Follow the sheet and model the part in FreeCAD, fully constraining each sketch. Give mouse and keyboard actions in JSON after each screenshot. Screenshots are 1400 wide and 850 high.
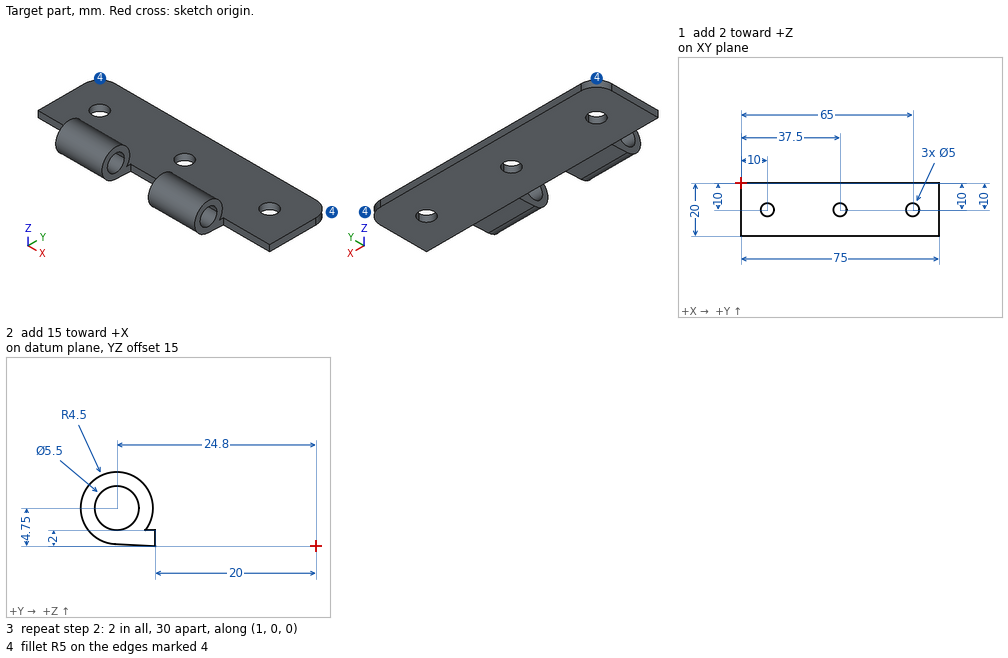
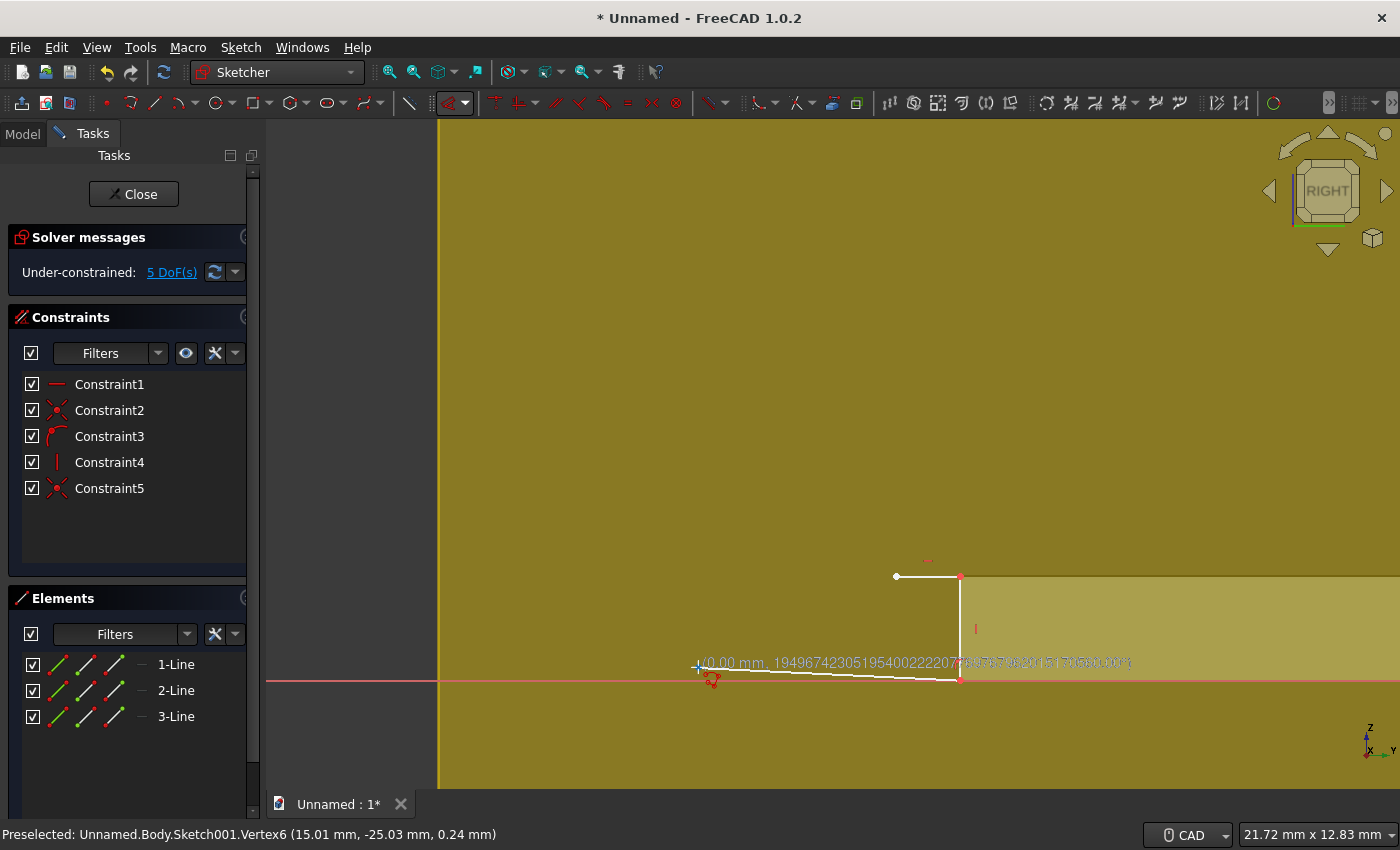
{"action": "key", "text": "g 3 a"}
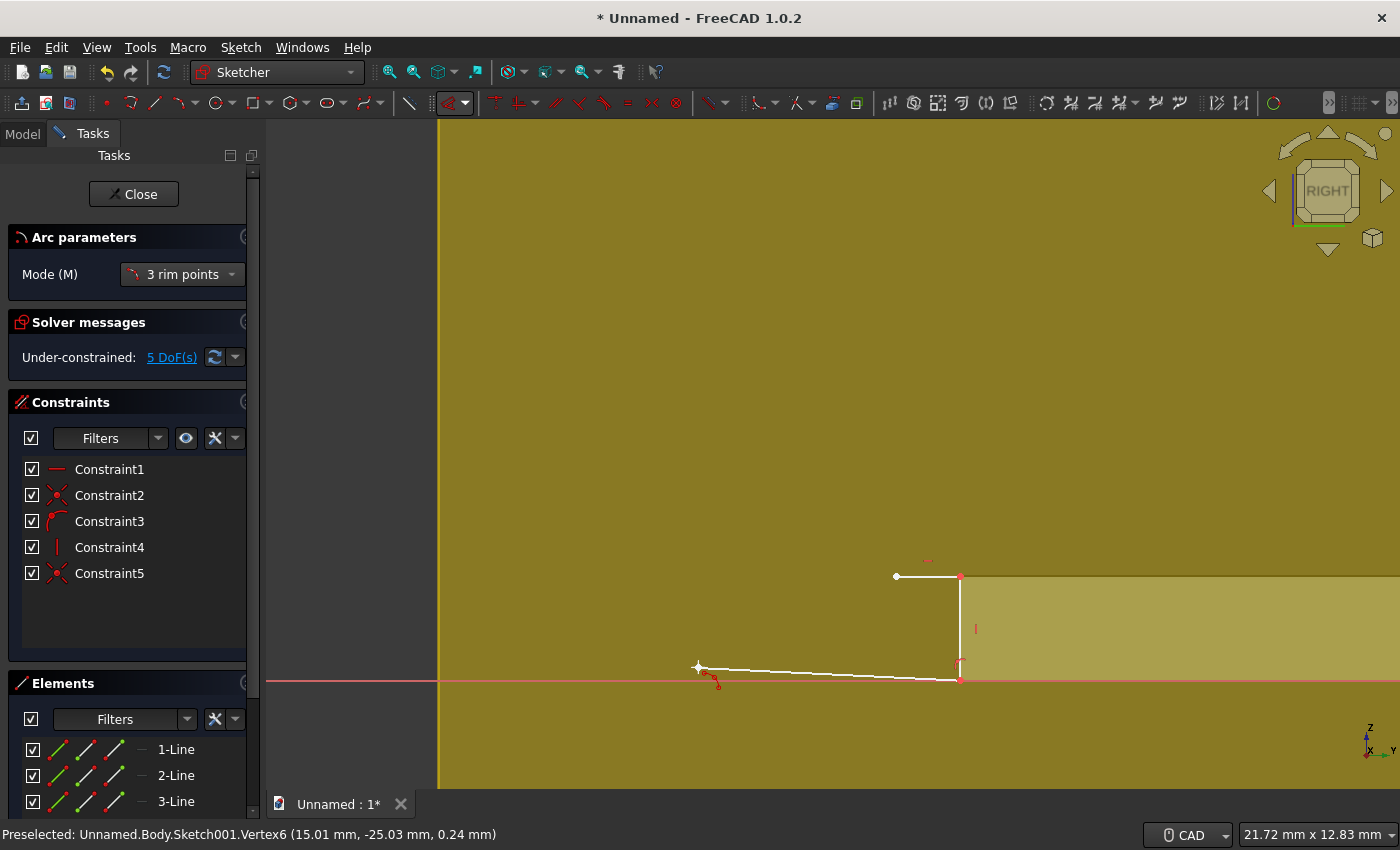
{"action": "left_click", "coordinate": [698, 668]}
{"action": "left_click", "coordinate": [896, 577]}
{"action": "left_click", "coordinate": [612, 219]}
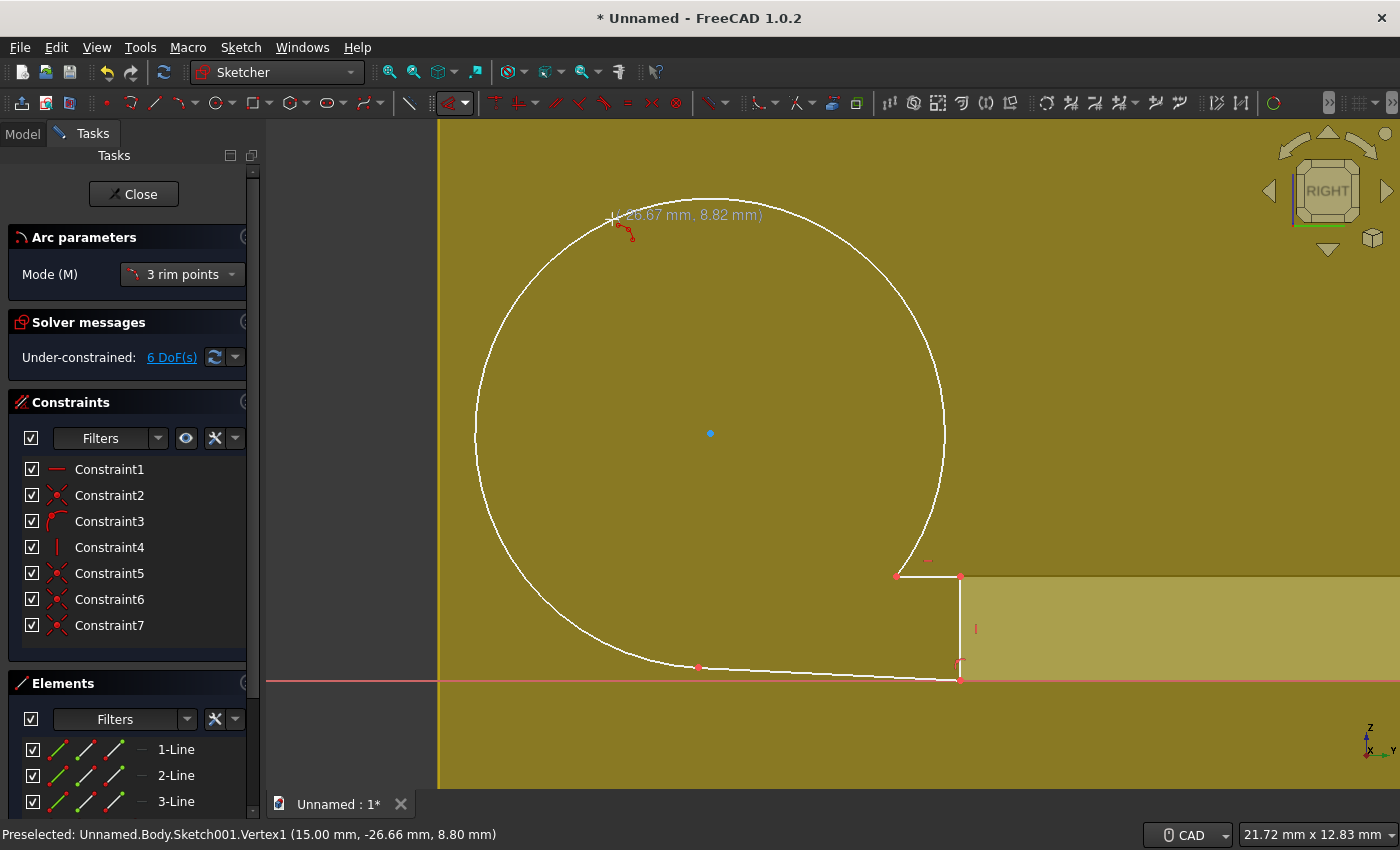
{"action": "key", "text": "g c"}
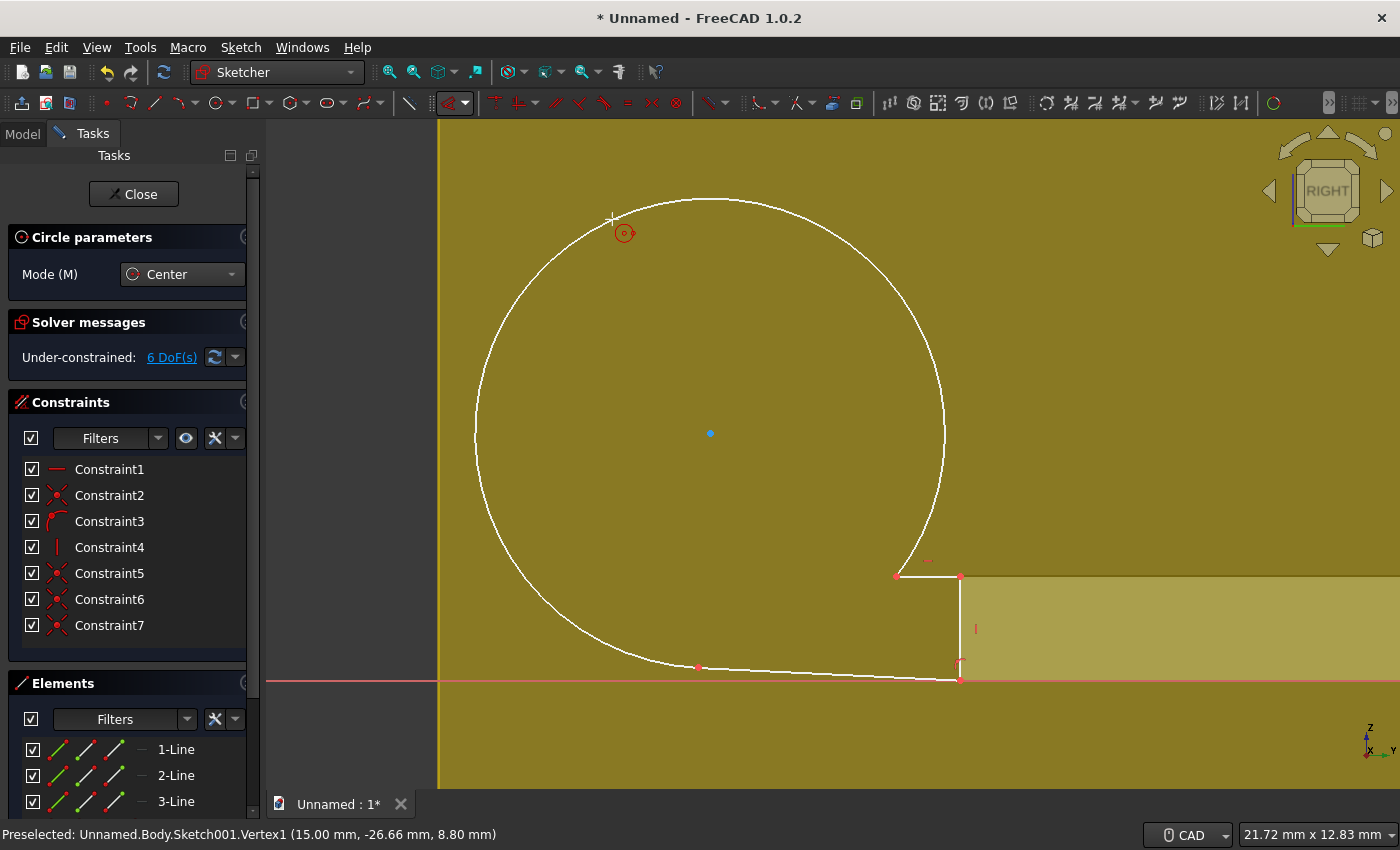
{"action": "left_click", "coordinate": [710, 433]}
{"action": "left_click", "coordinate": [811, 331]}
{"action": "key", "text": "Escape"}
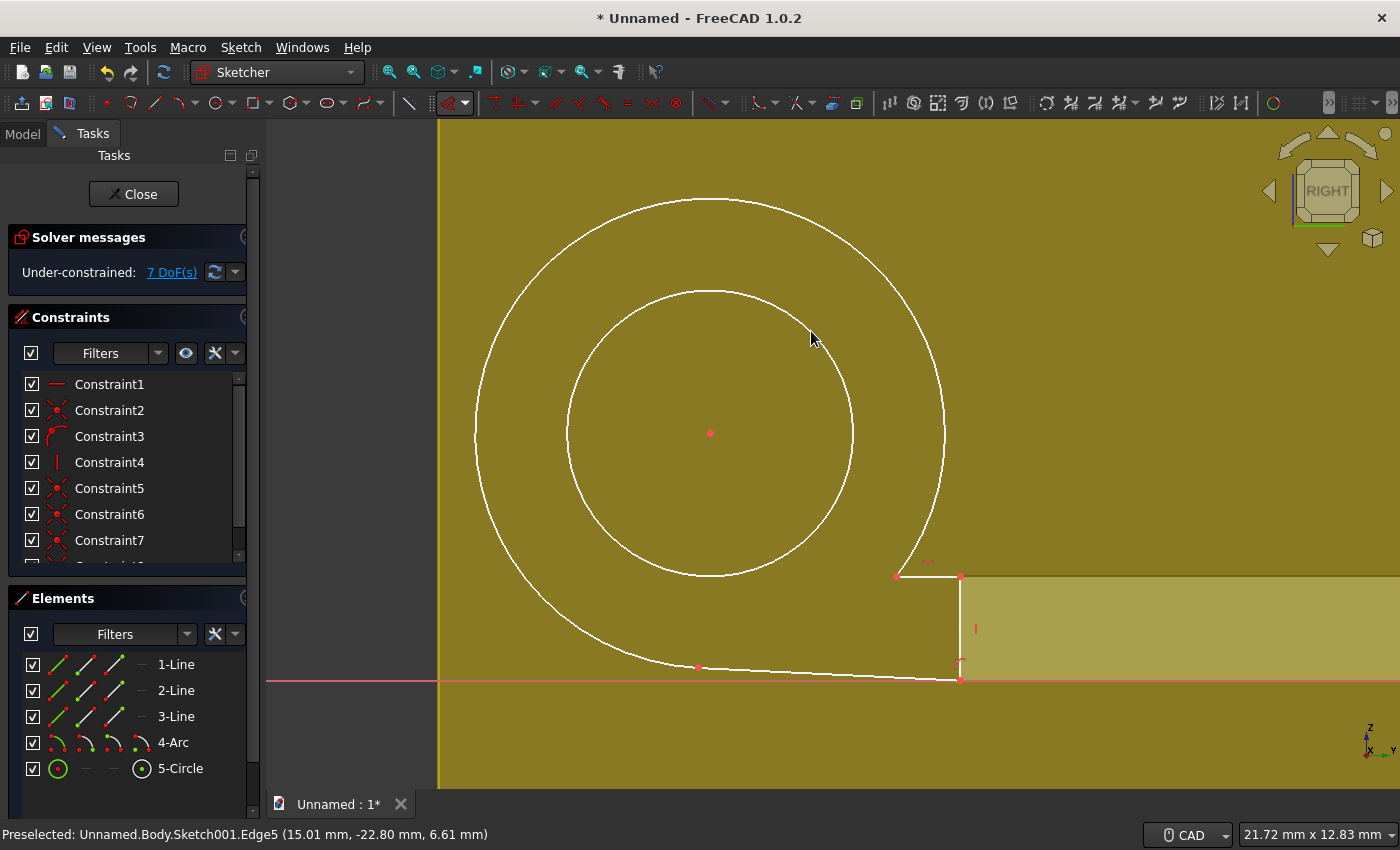
{"action": "left_click", "coordinate": [881, 677]}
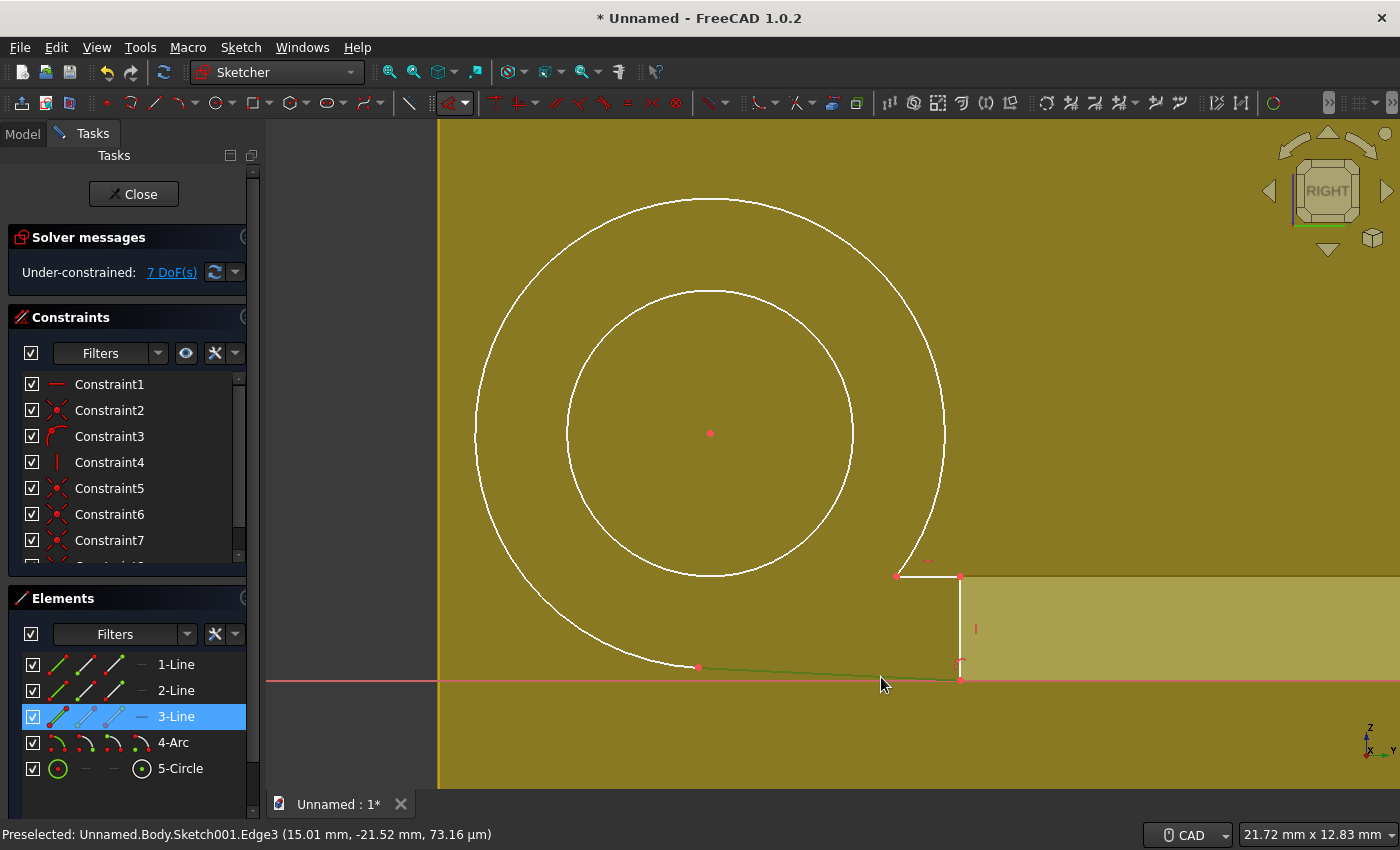
{"action": "left_click", "coordinate": [849, 244]}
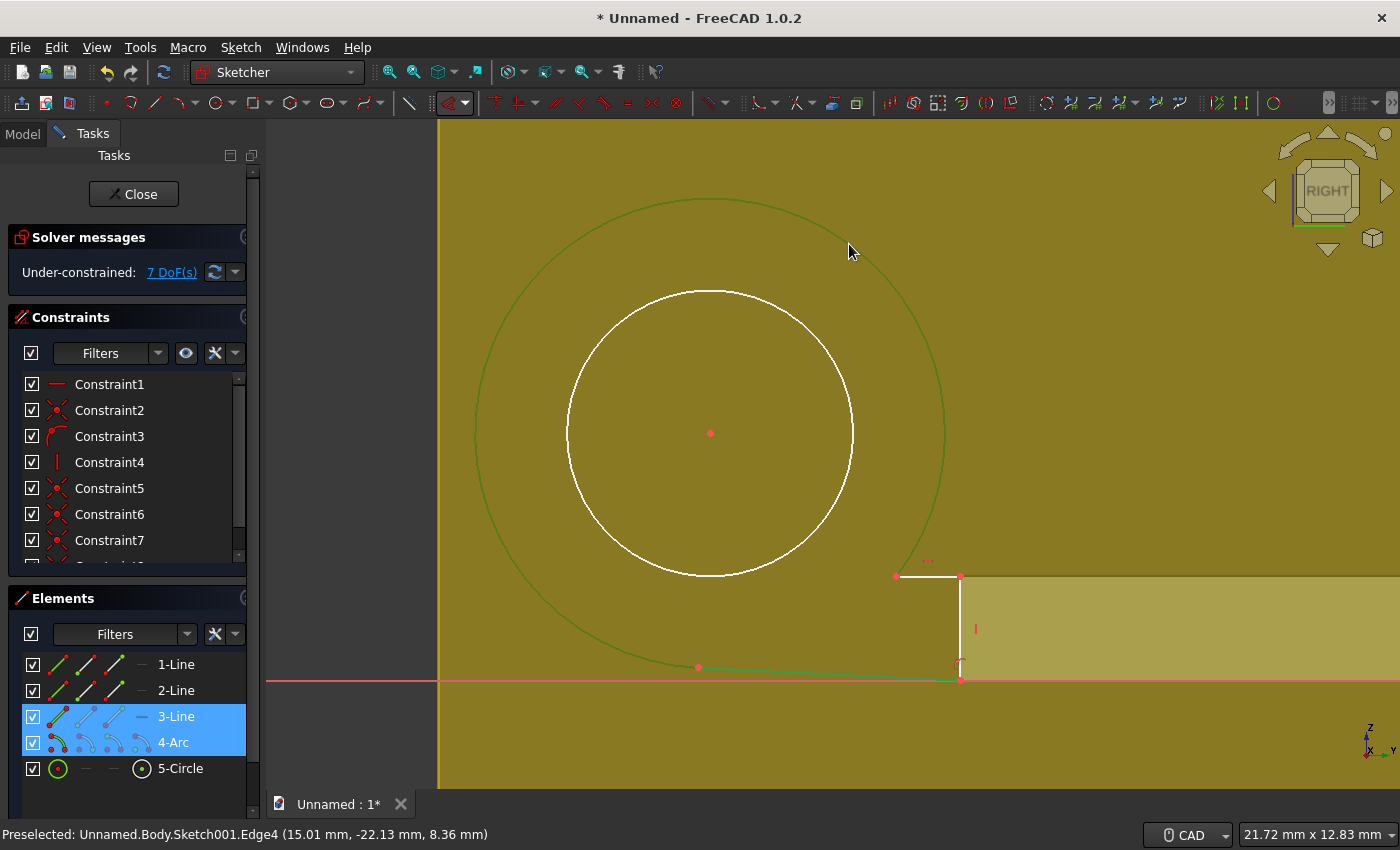
{"action": "key", "text": "t"}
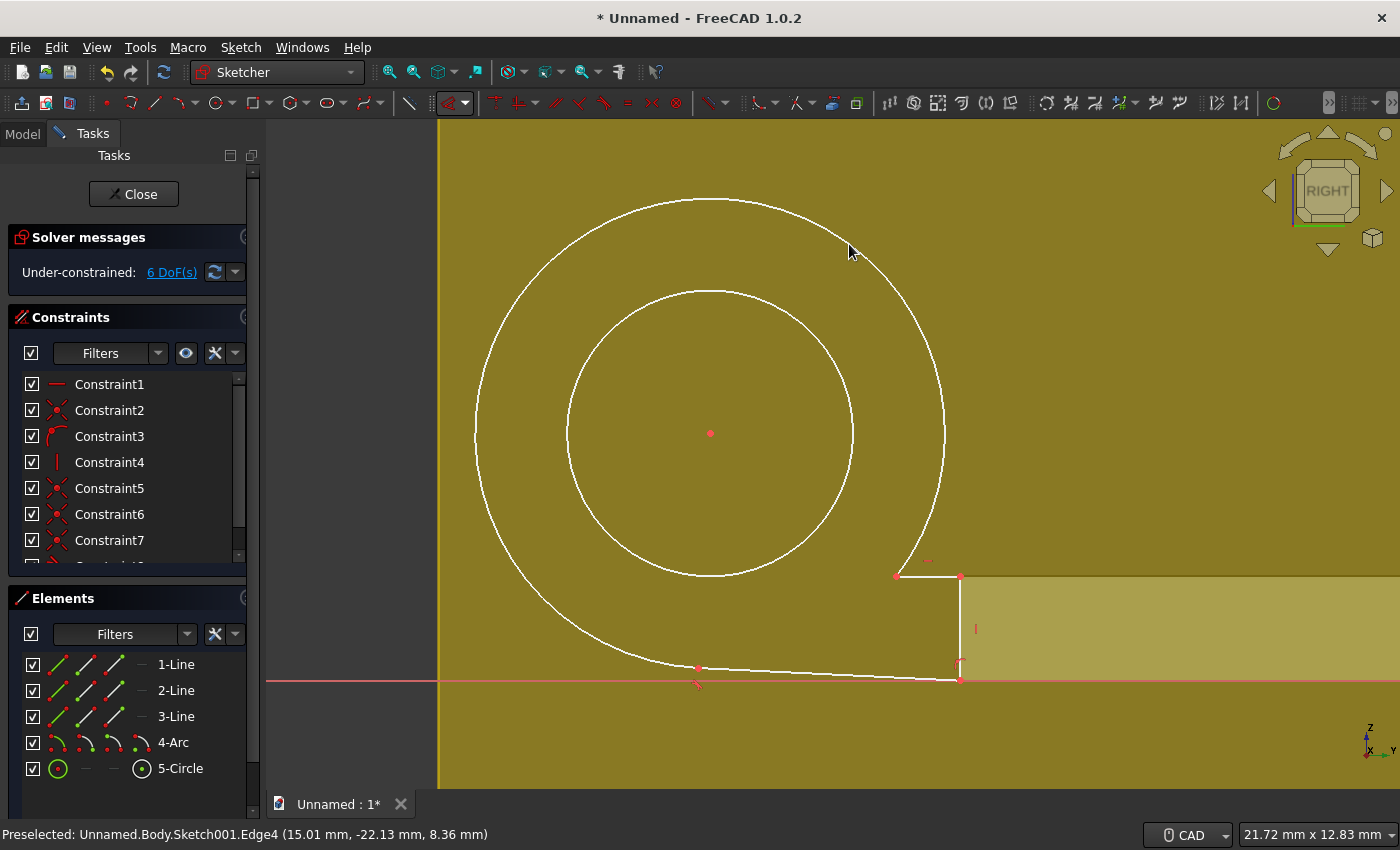
{"action": "left_click", "coordinate": [849, 244]}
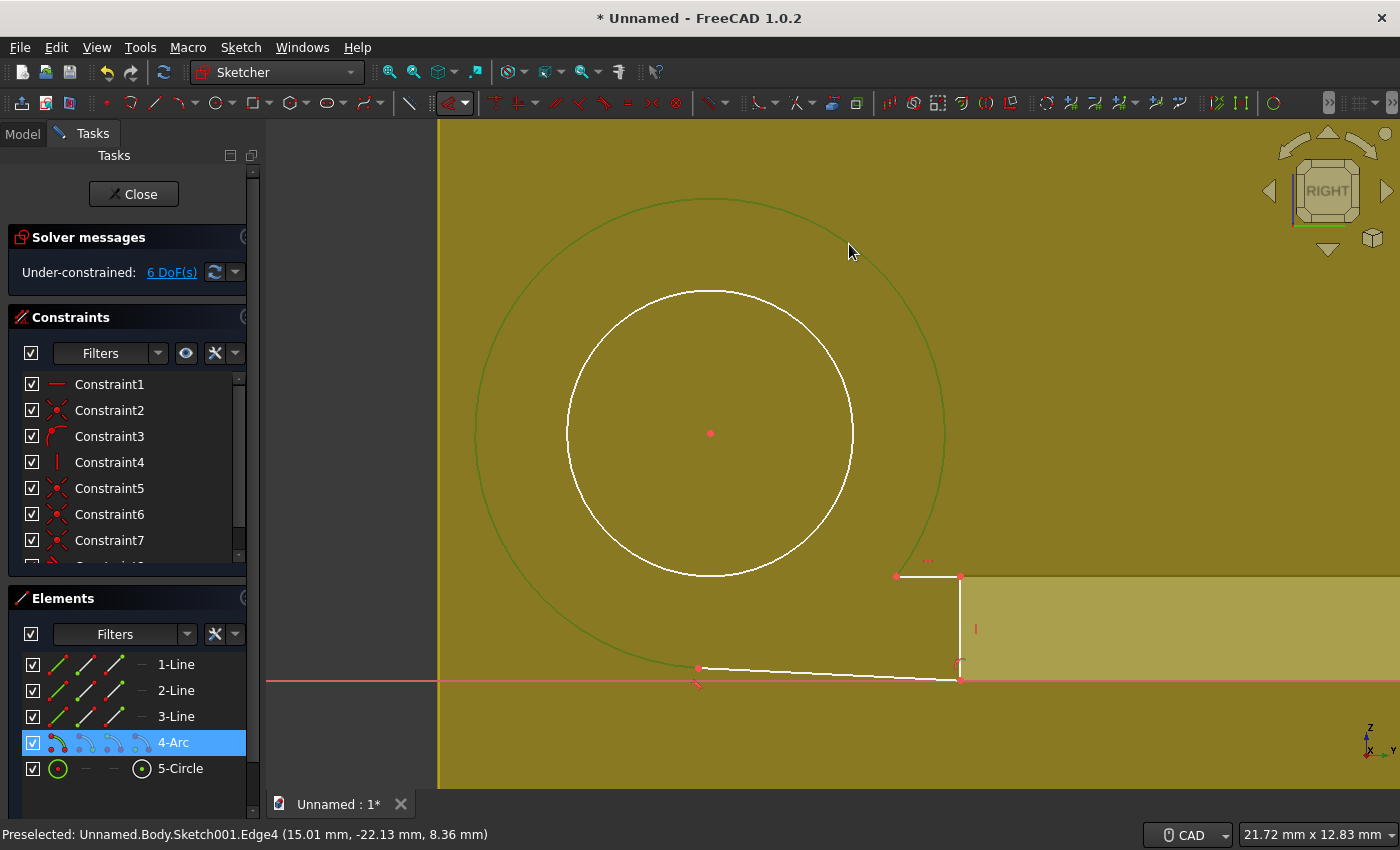
{"action": "key", "text": "k r"}